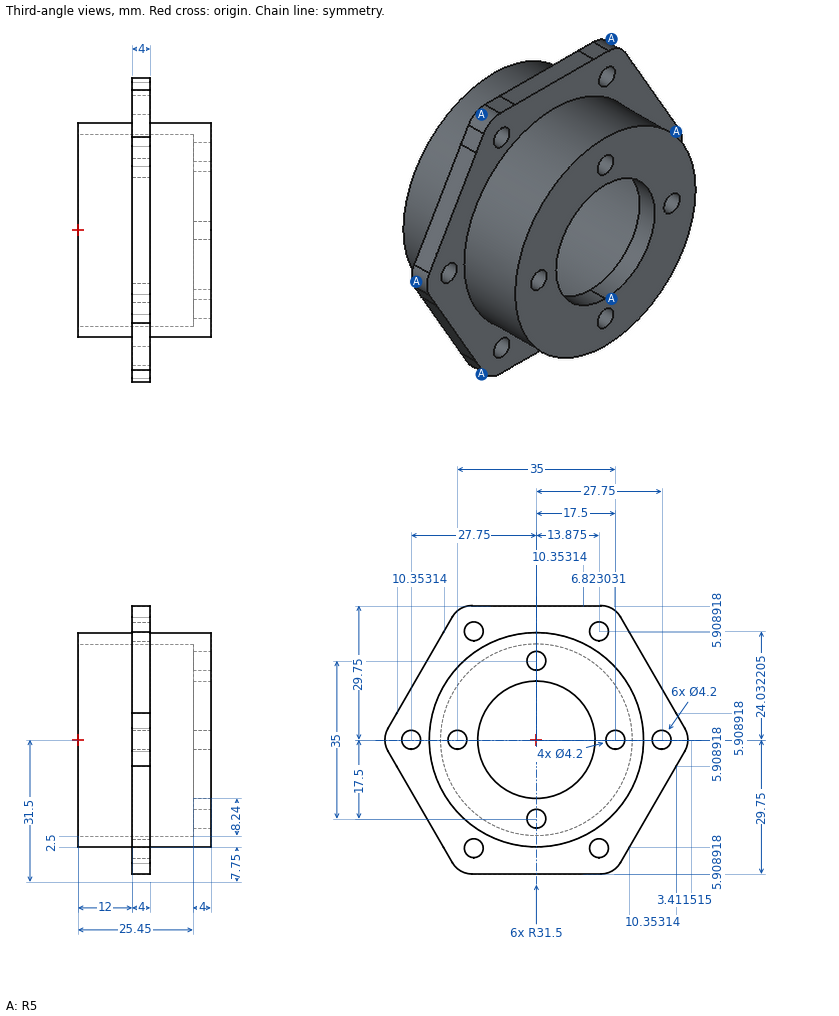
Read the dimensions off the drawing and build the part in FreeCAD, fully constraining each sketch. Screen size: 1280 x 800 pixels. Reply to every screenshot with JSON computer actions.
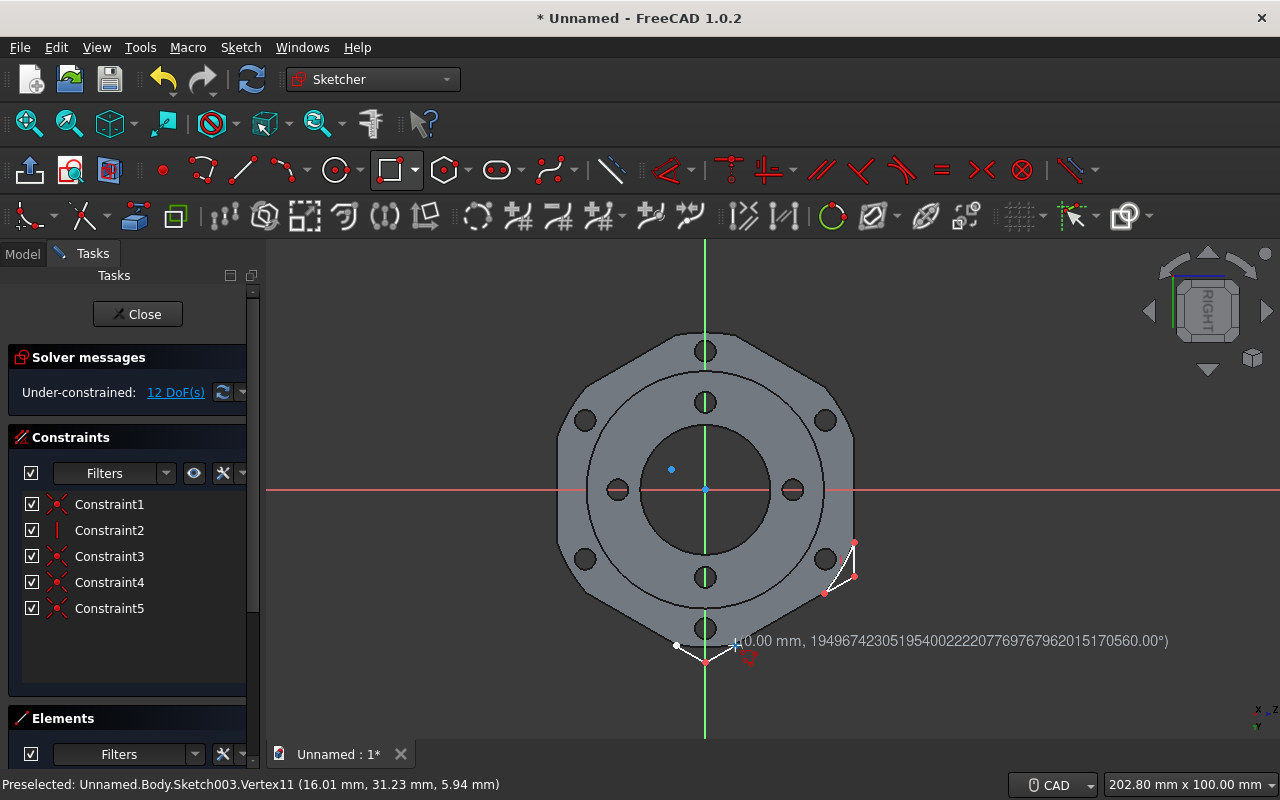
{"action": "left_click", "coordinate": [284, 170]}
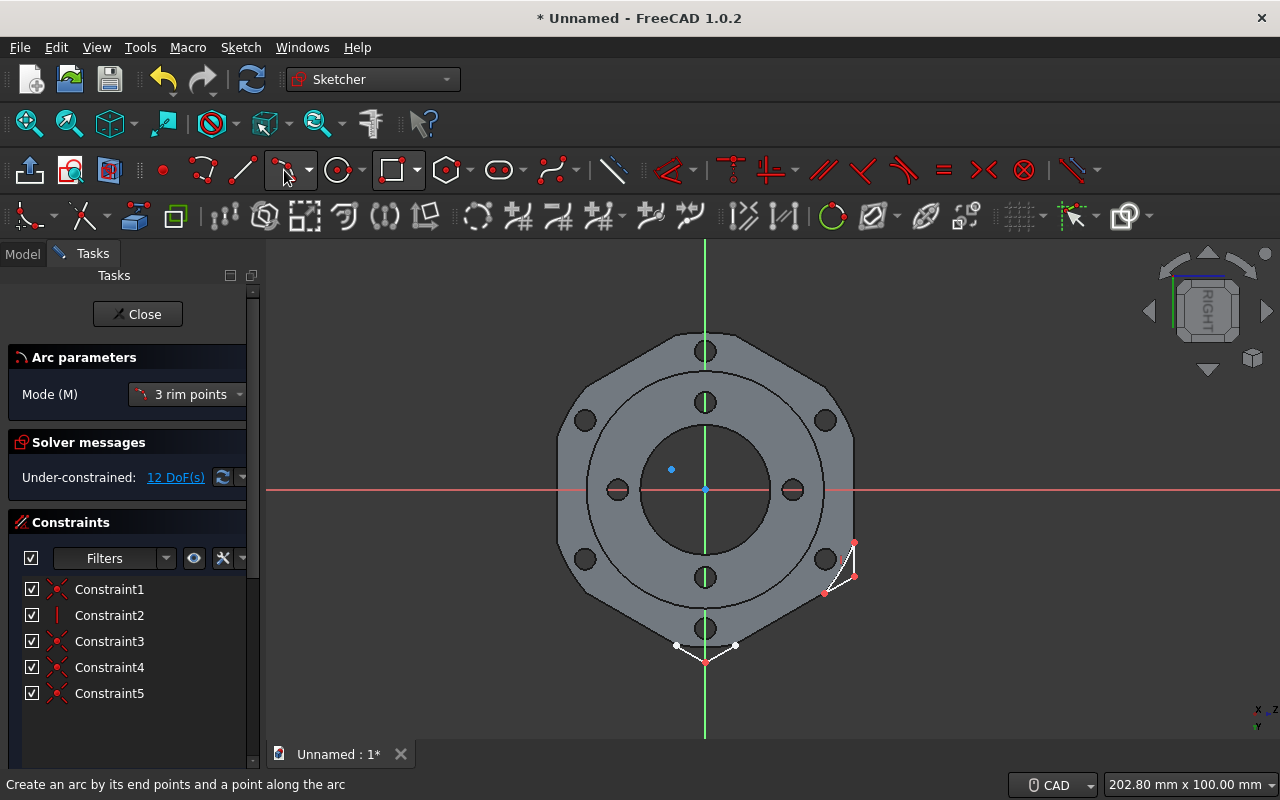
{"action": "left_click", "coordinate": [735, 646]}
{"action": "left_click", "coordinate": [676, 646]}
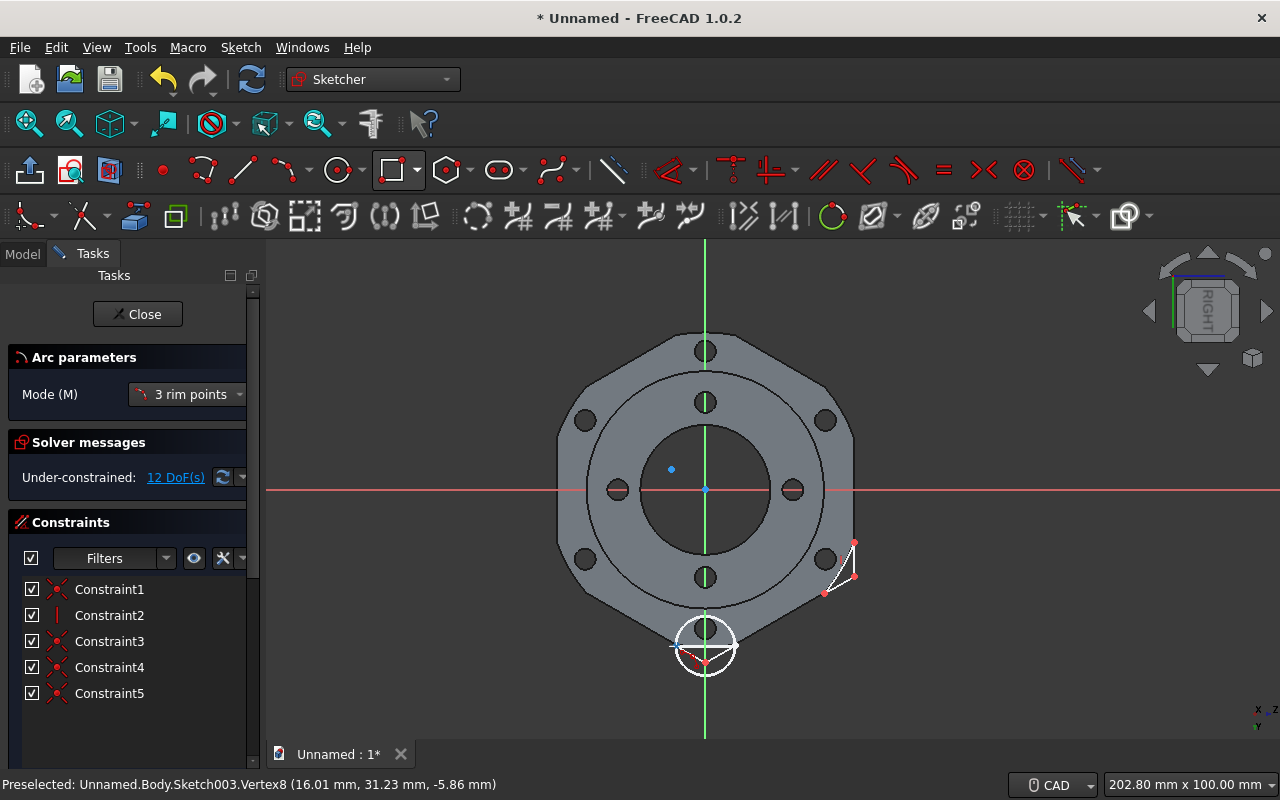
{"action": "scroll", "coordinate": [699, 647], "scroll_direction": "up", "scroll_amount": 9}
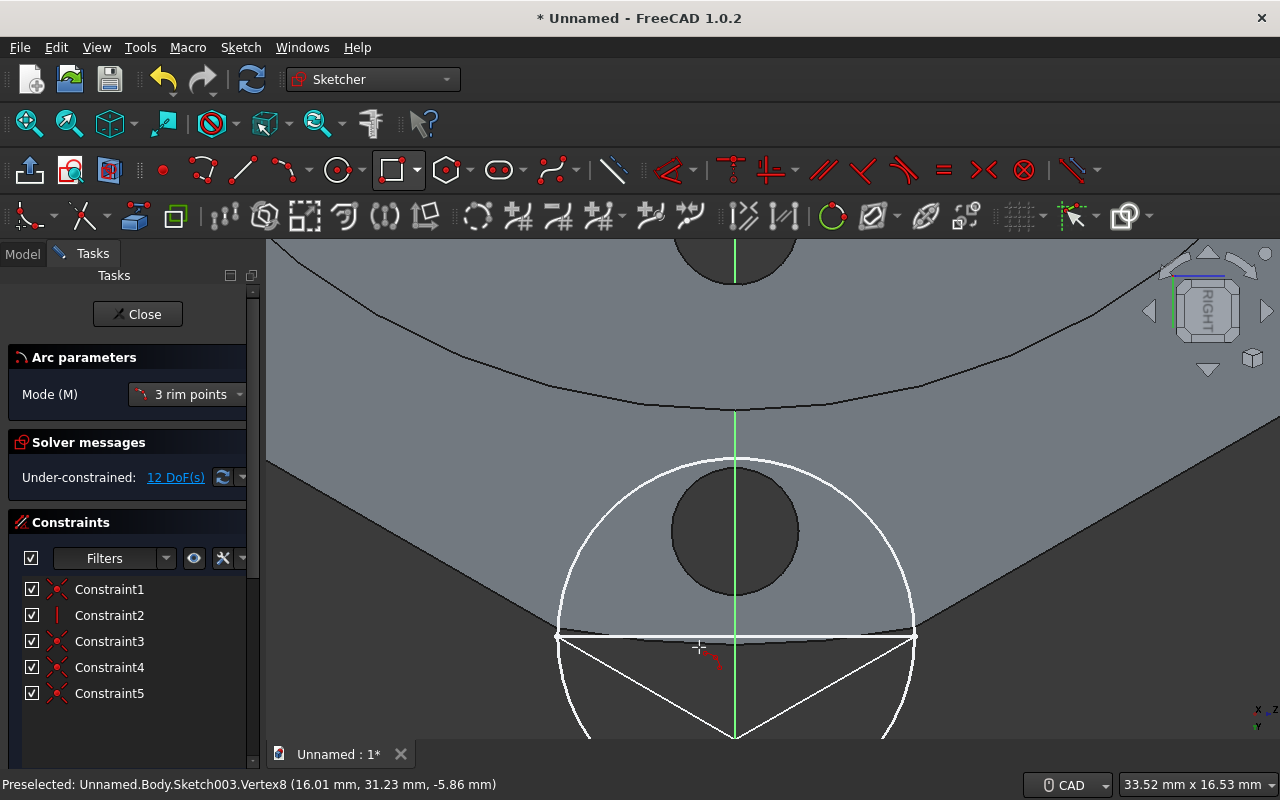
{"action": "left_click", "coordinate": [699, 644]}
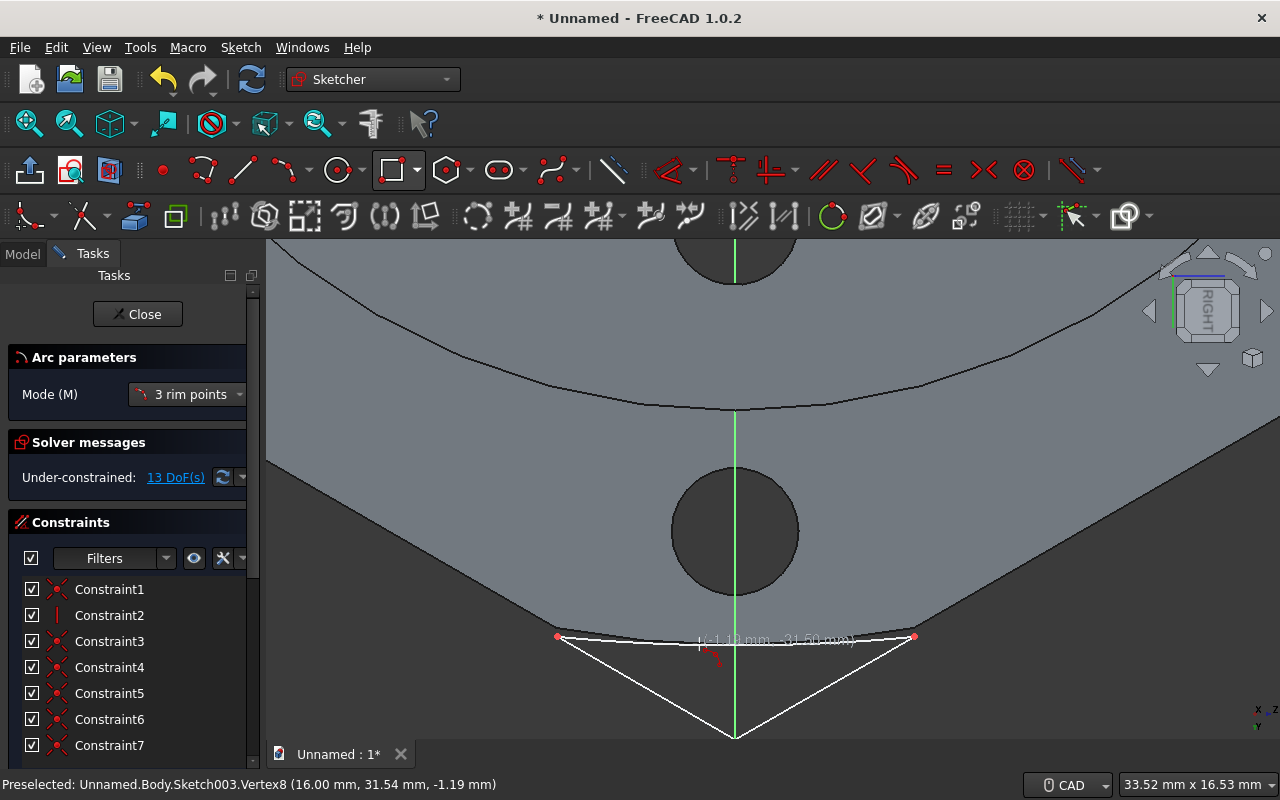
{"action": "key", "text": "g m"}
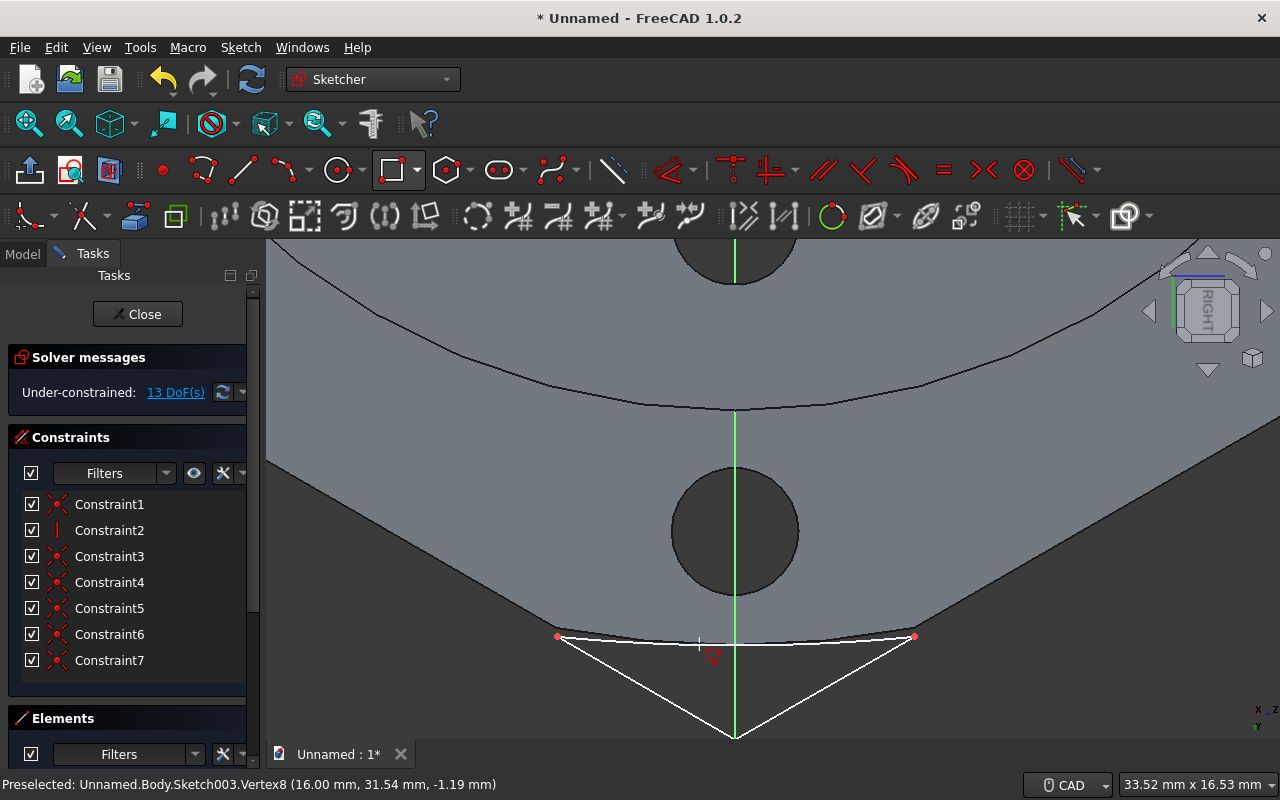
{"action": "scroll", "coordinate": [698, 647], "scroll_direction": "down", "scroll_amount": 9}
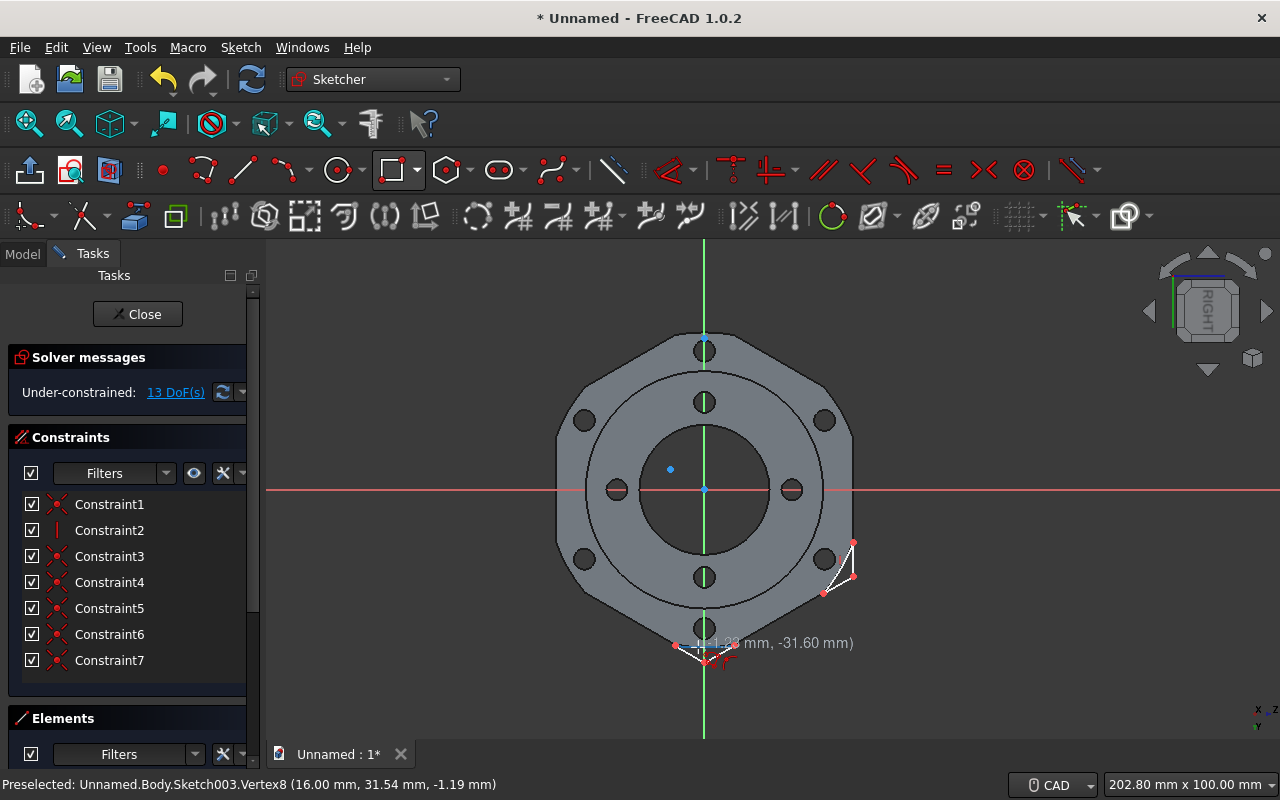
{"action": "left_click", "coordinate": [556, 542]}
{"action": "left_click", "coordinate": [556, 576]}
{"action": "left_click", "coordinate": [585, 593]}
{"action": "right_click", "coordinate": [585, 593]}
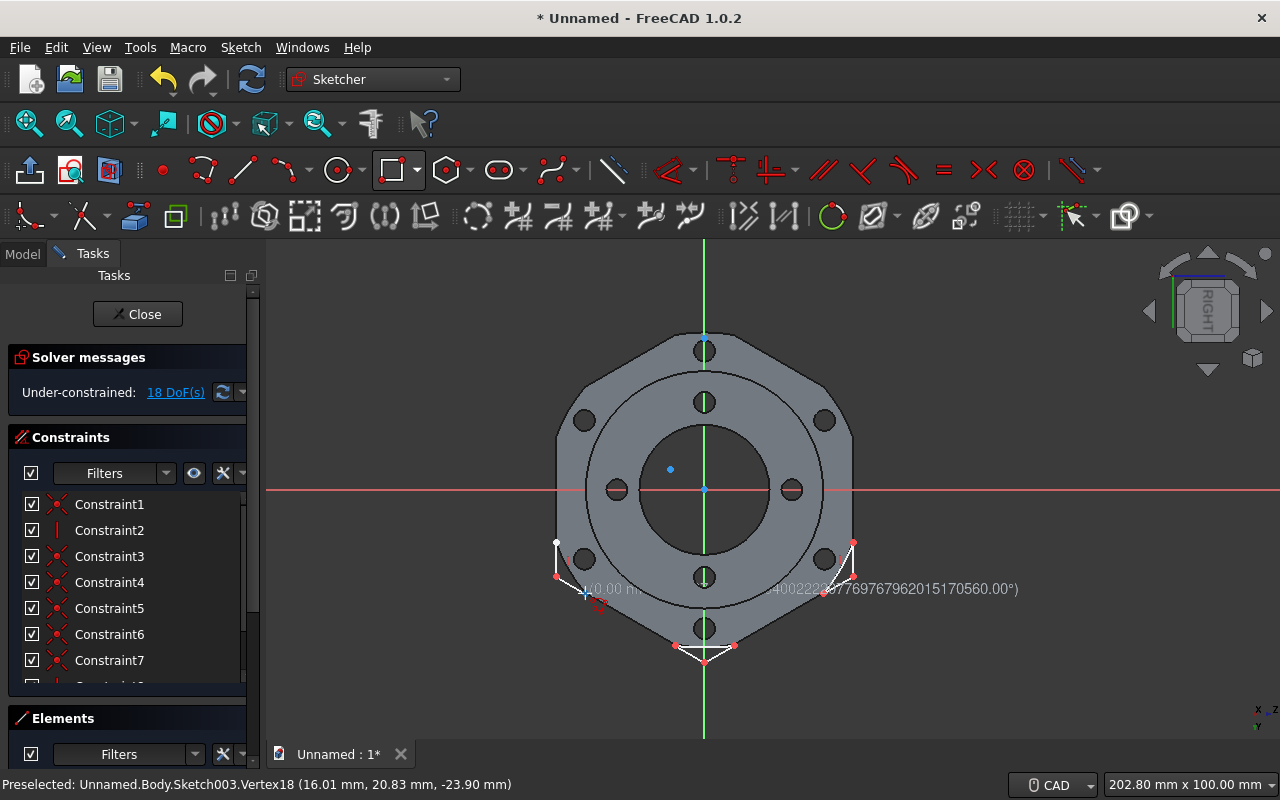
{"action": "key", "text": "g 3 a"}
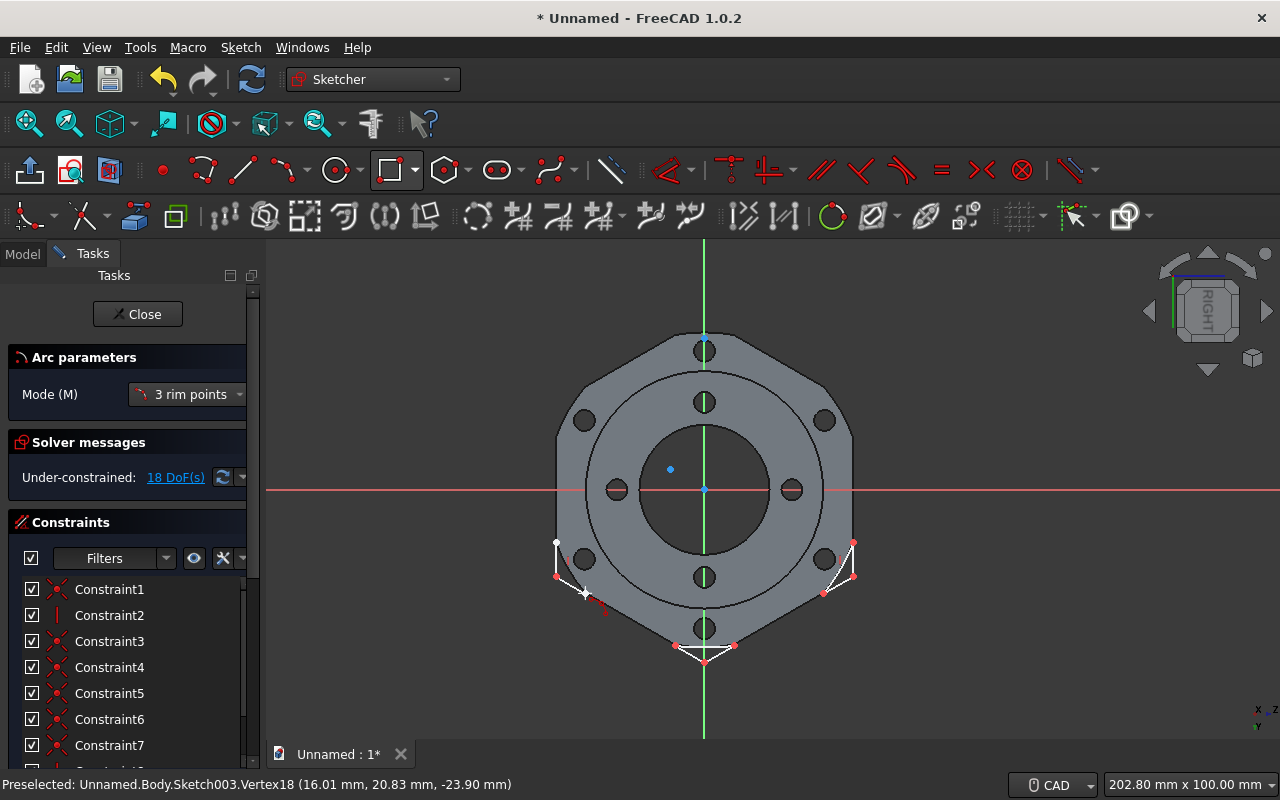
{"action": "left_click", "coordinate": [585, 594]}
{"action": "left_click", "coordinate": [556, 543]}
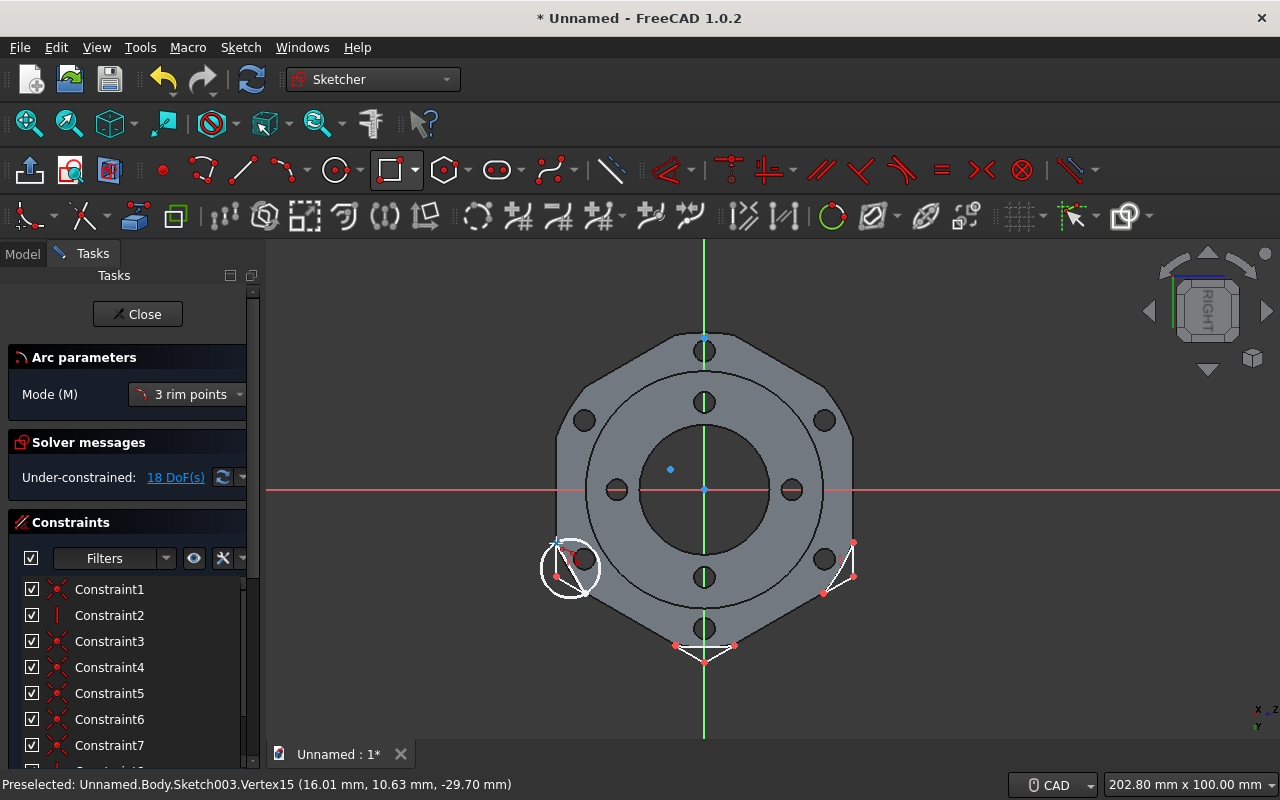
{"action": "scroll", "coordinate": [568, 569], "scroll_direction": "up", "scroll_amount": 9}